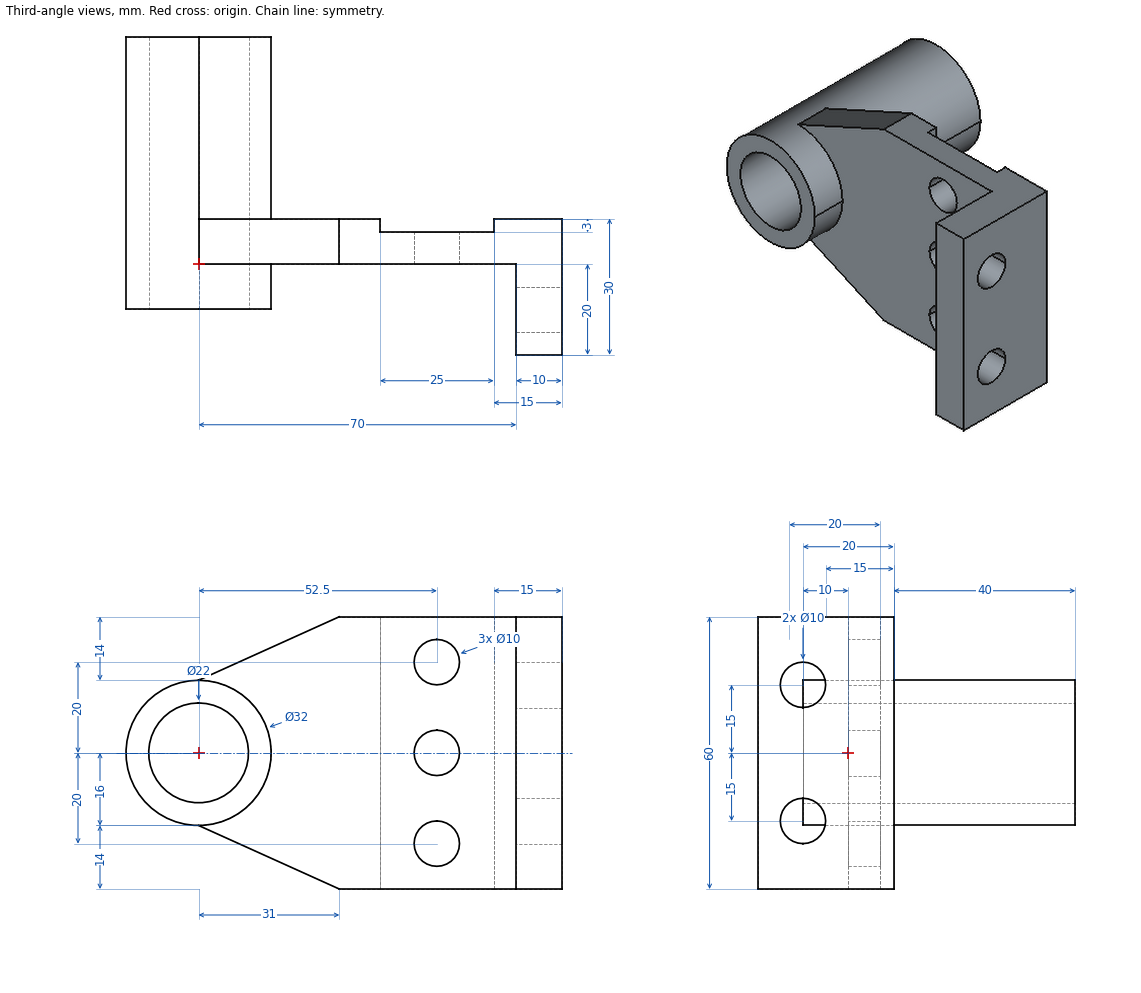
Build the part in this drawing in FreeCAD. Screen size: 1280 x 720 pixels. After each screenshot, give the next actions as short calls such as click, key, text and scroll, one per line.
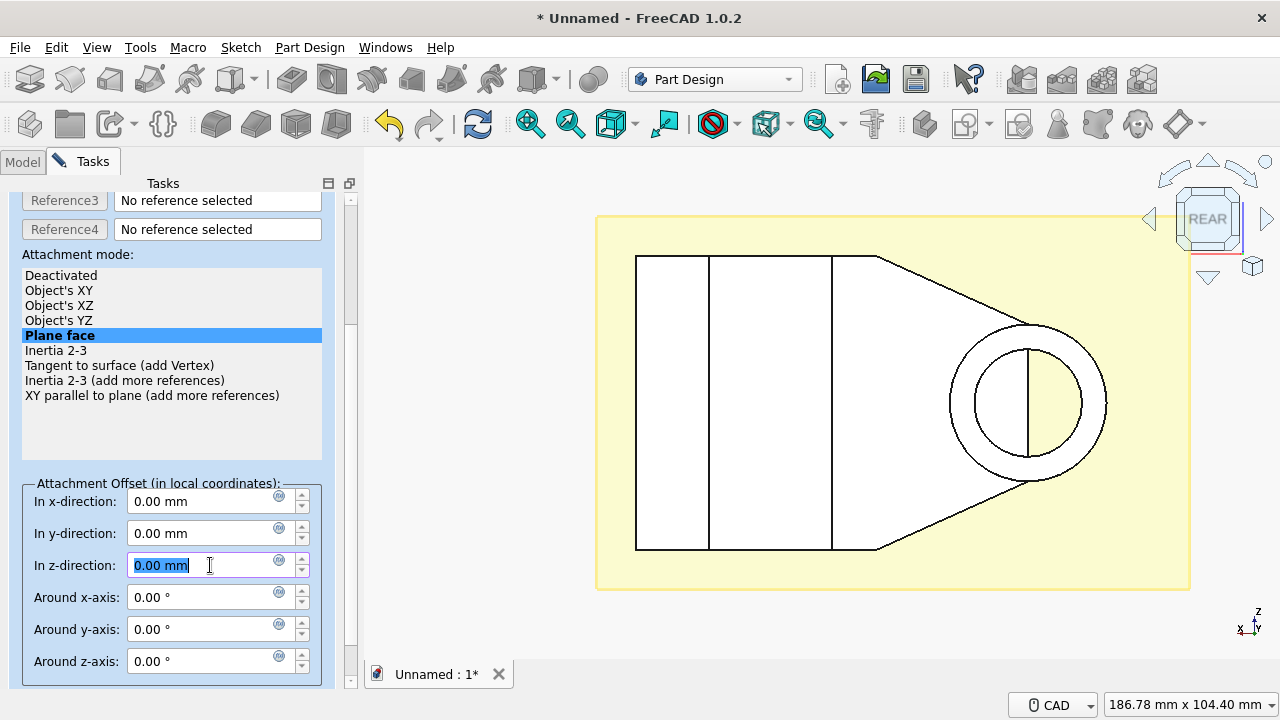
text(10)
key(Tab)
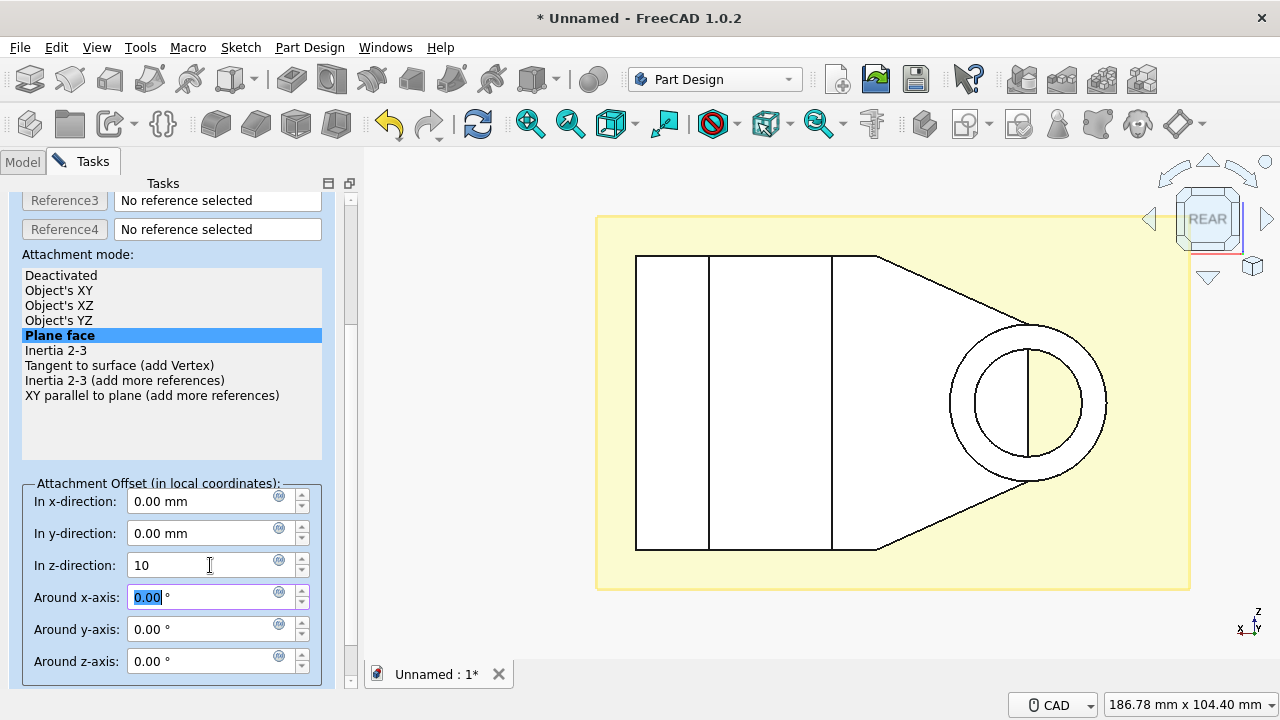
scroll(351, 440, up, 4)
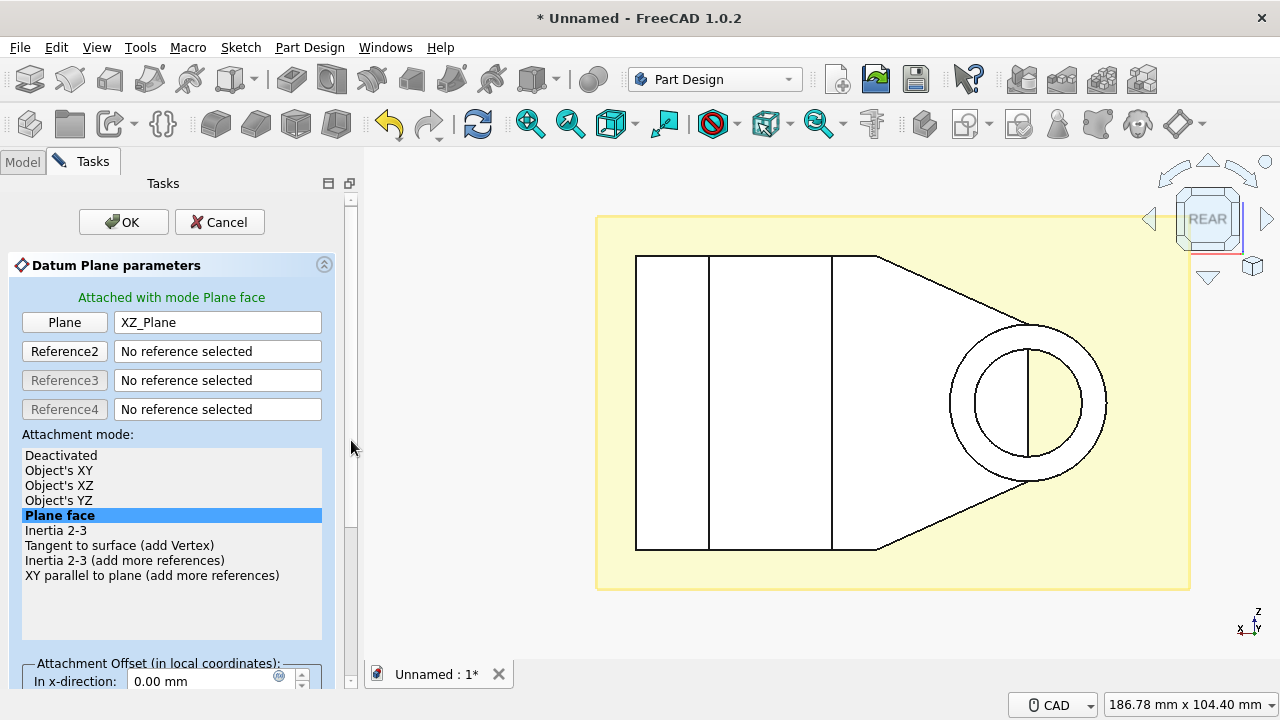
click(124, 222)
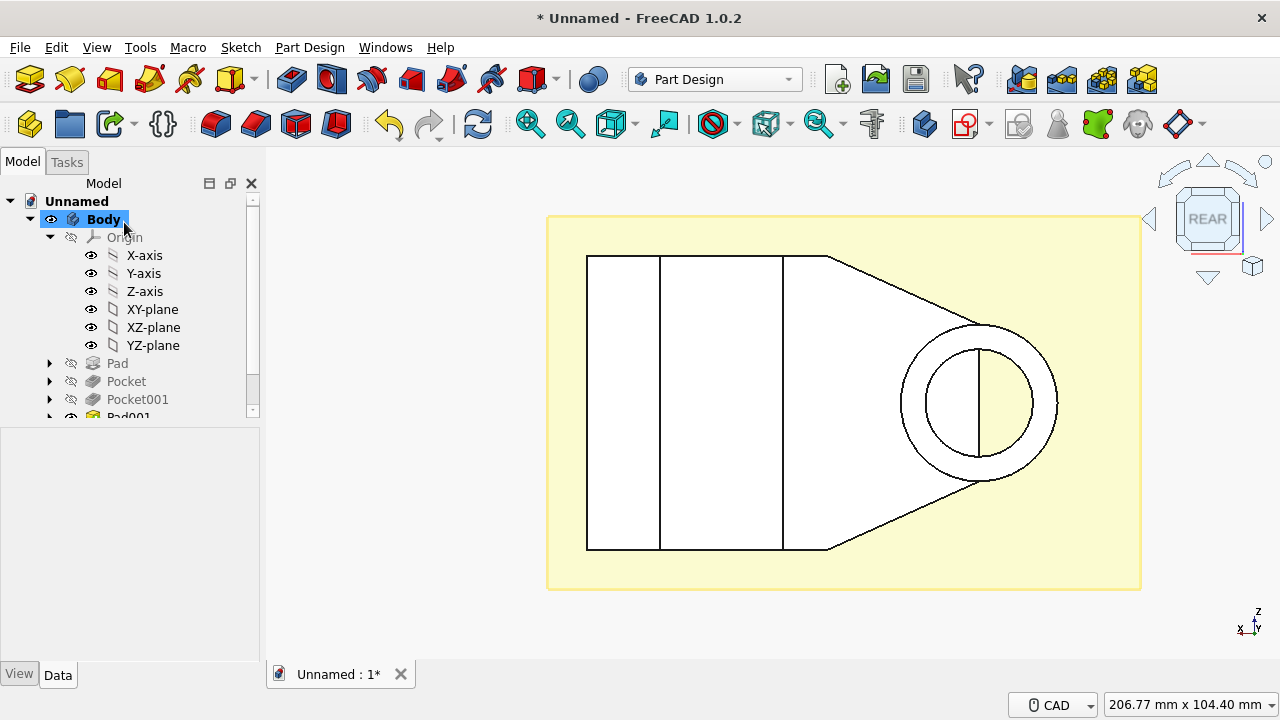
scroll(100, 305, down, 3)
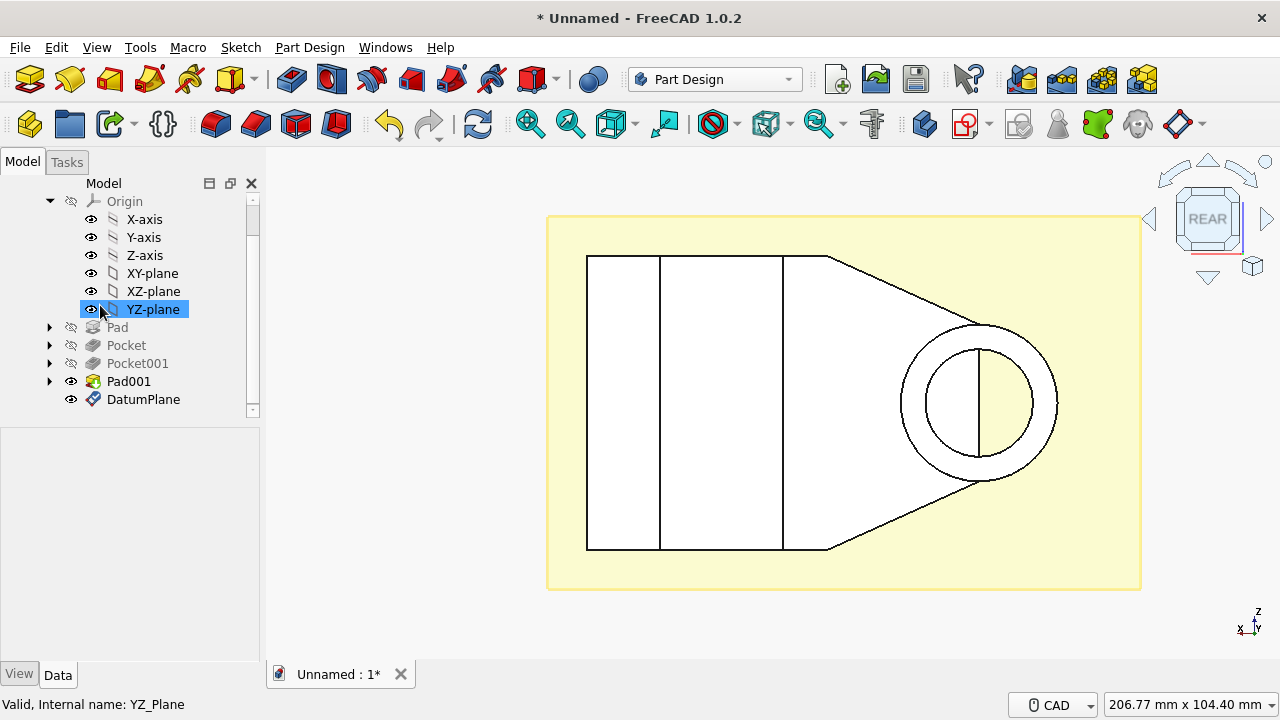
click(116, 399)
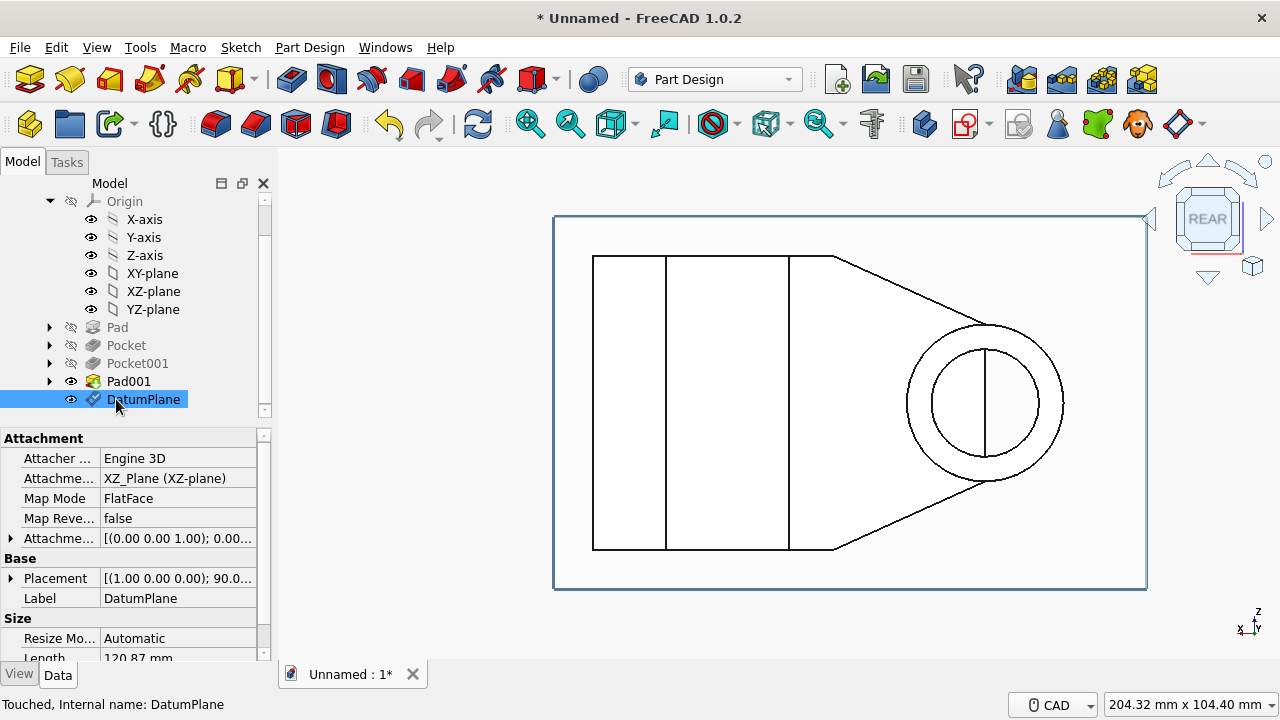
click(966, 124)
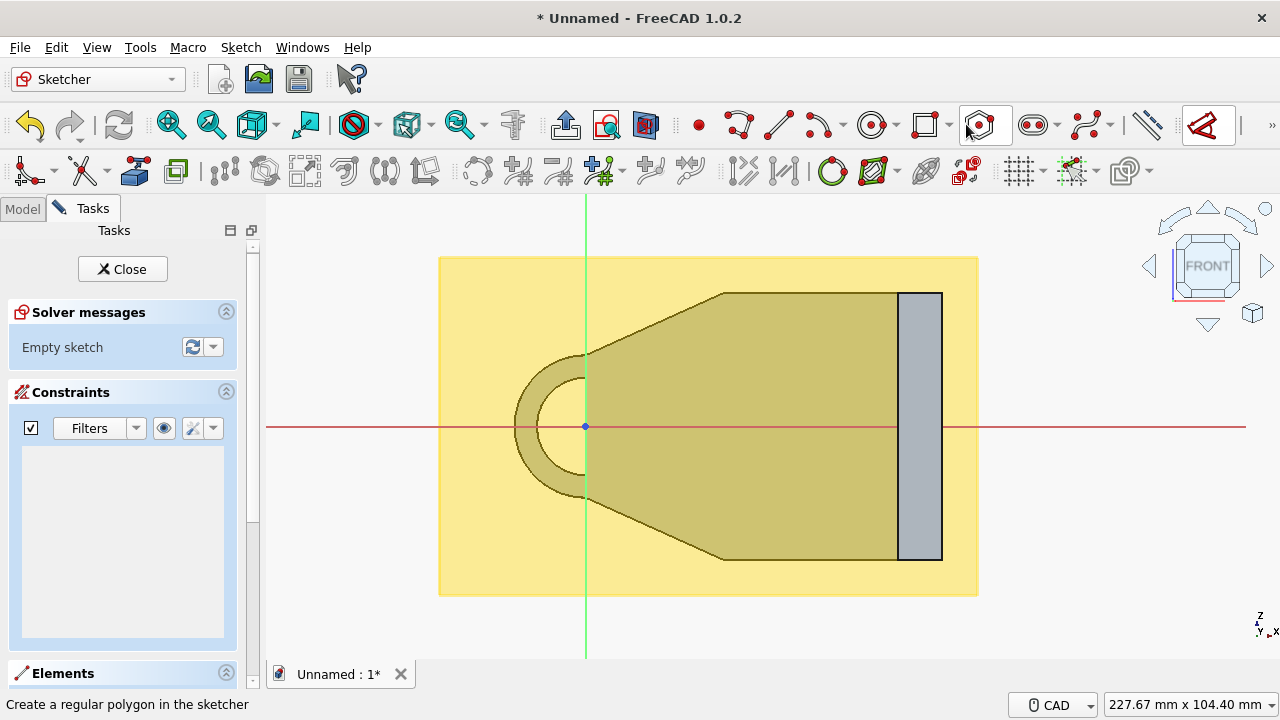
click(646, 126)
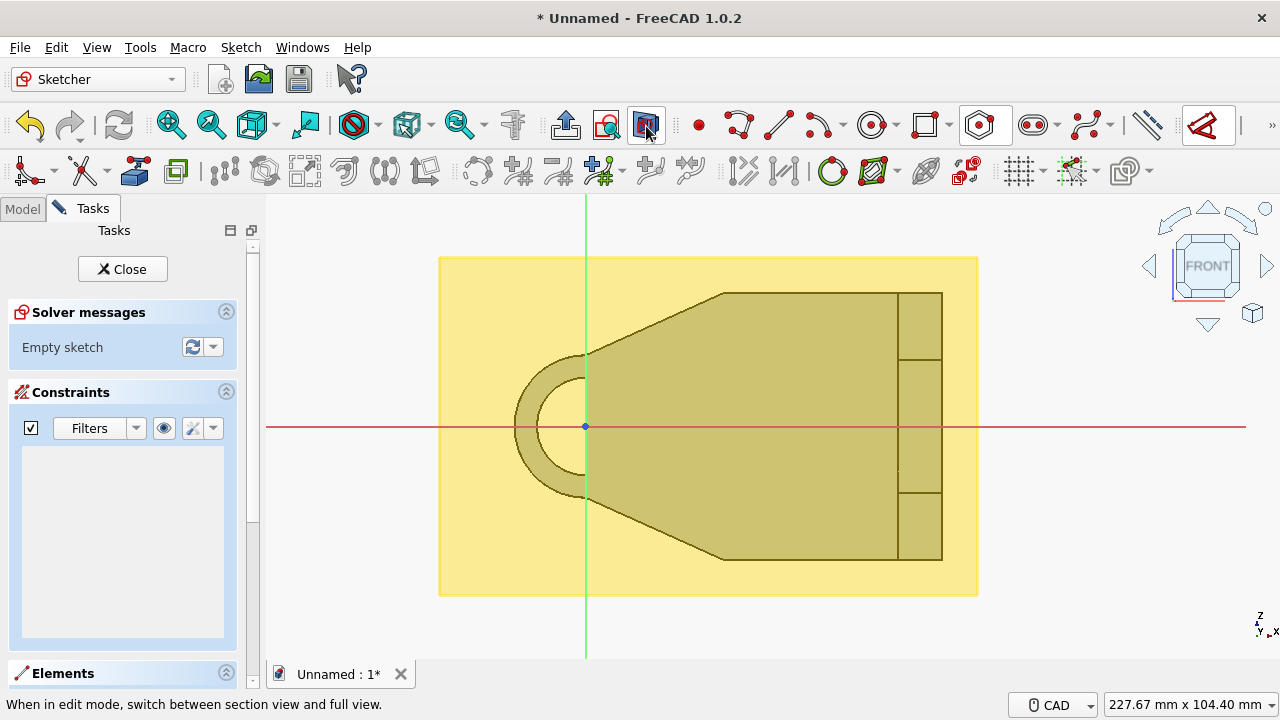
scroll(489, 427, up, 4)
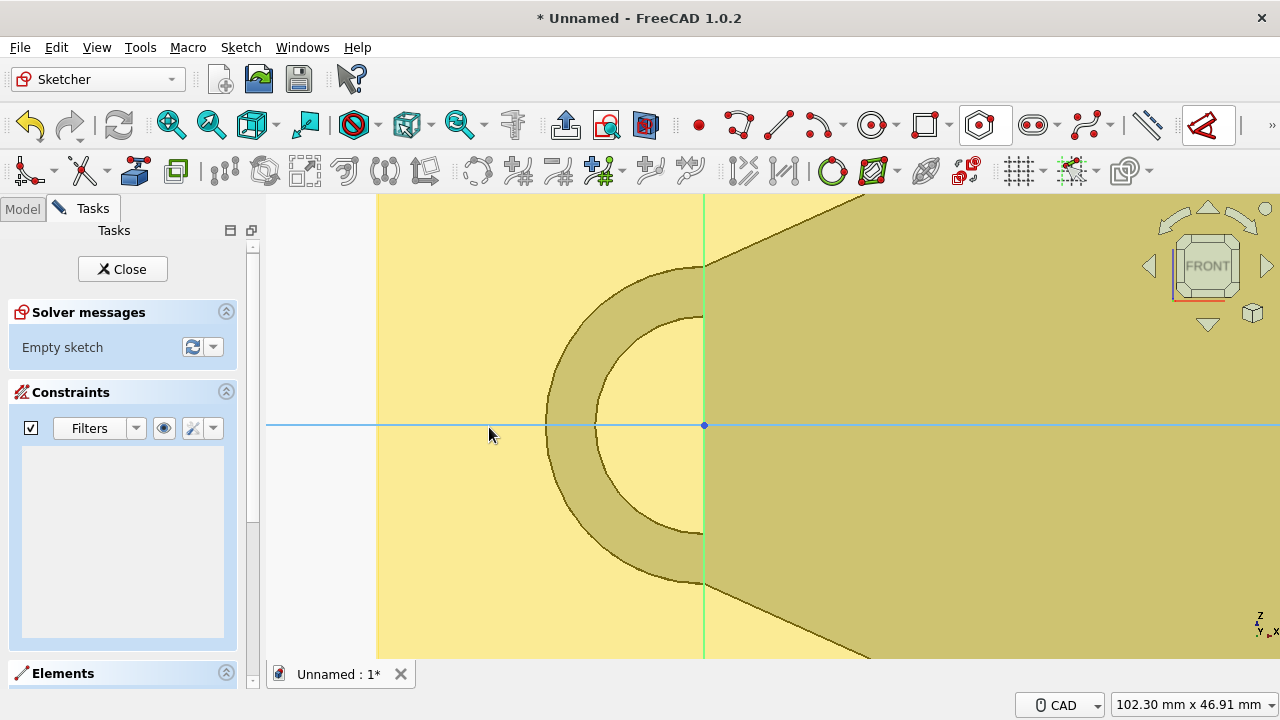
click(872, 126)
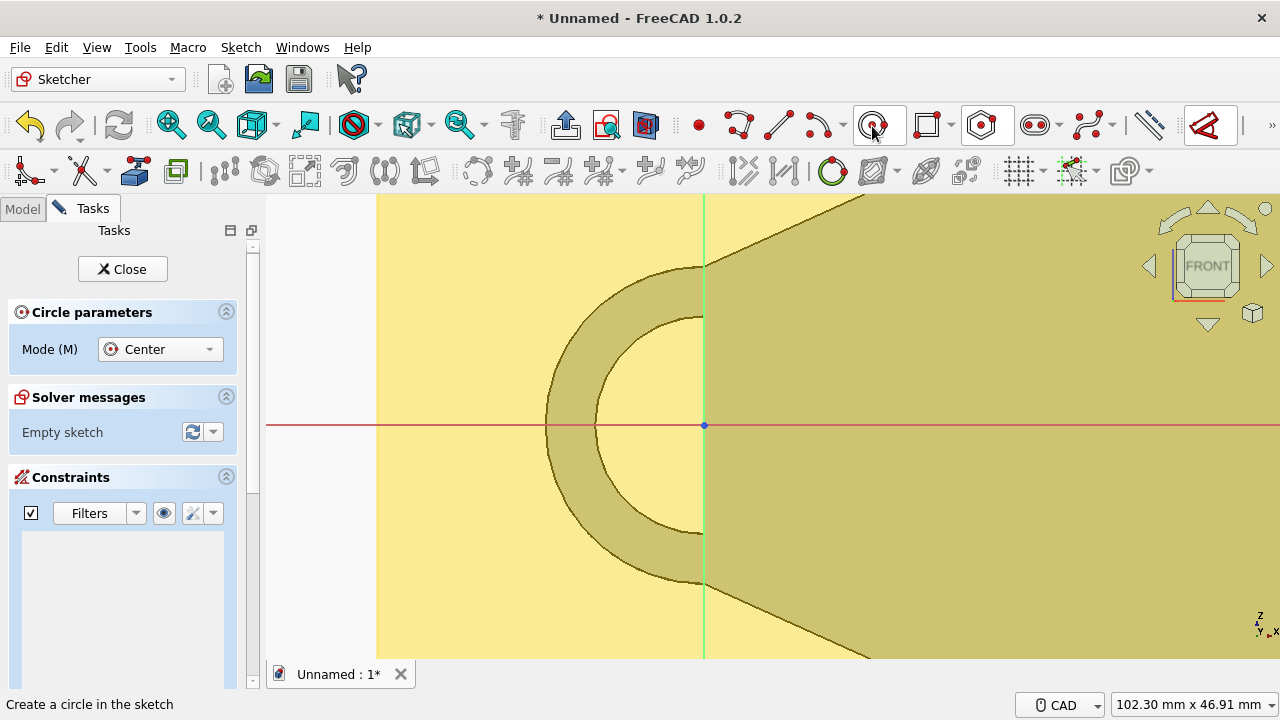
click(704, 425)
move(816, 313)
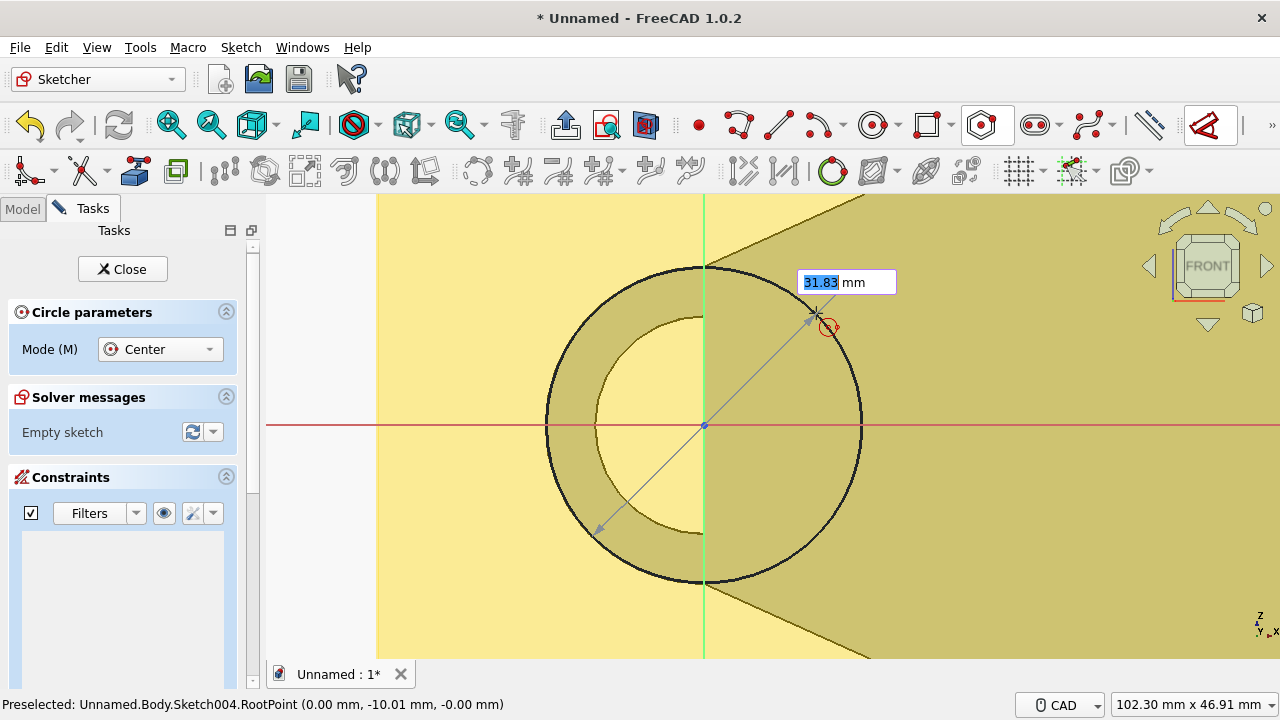
text(32)
key(Return)